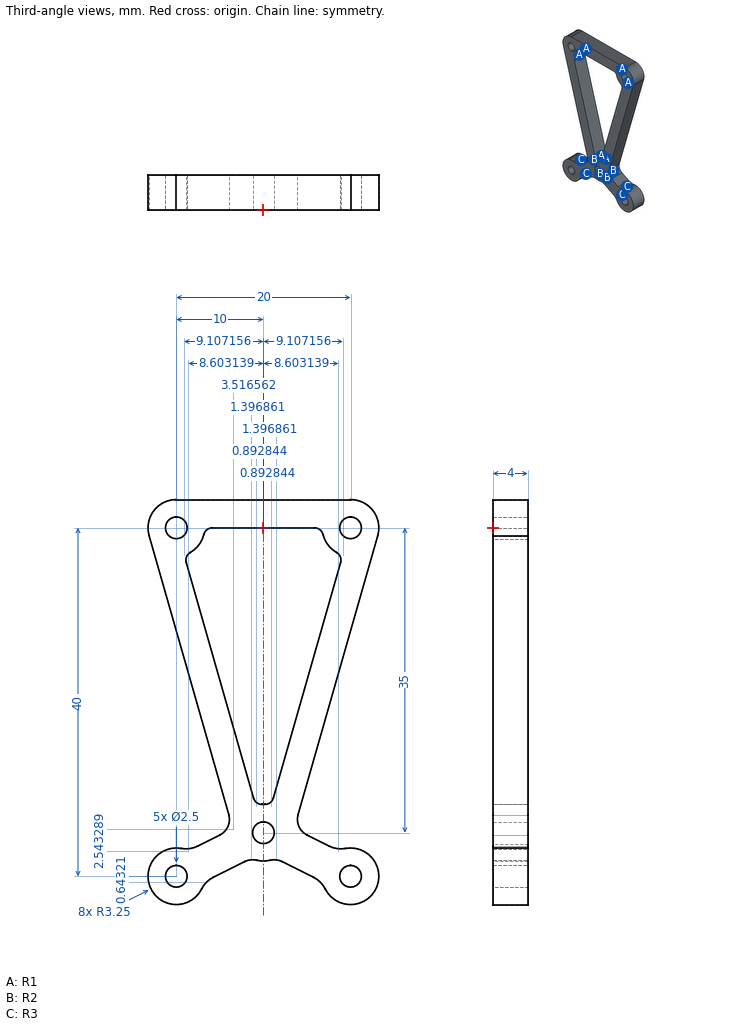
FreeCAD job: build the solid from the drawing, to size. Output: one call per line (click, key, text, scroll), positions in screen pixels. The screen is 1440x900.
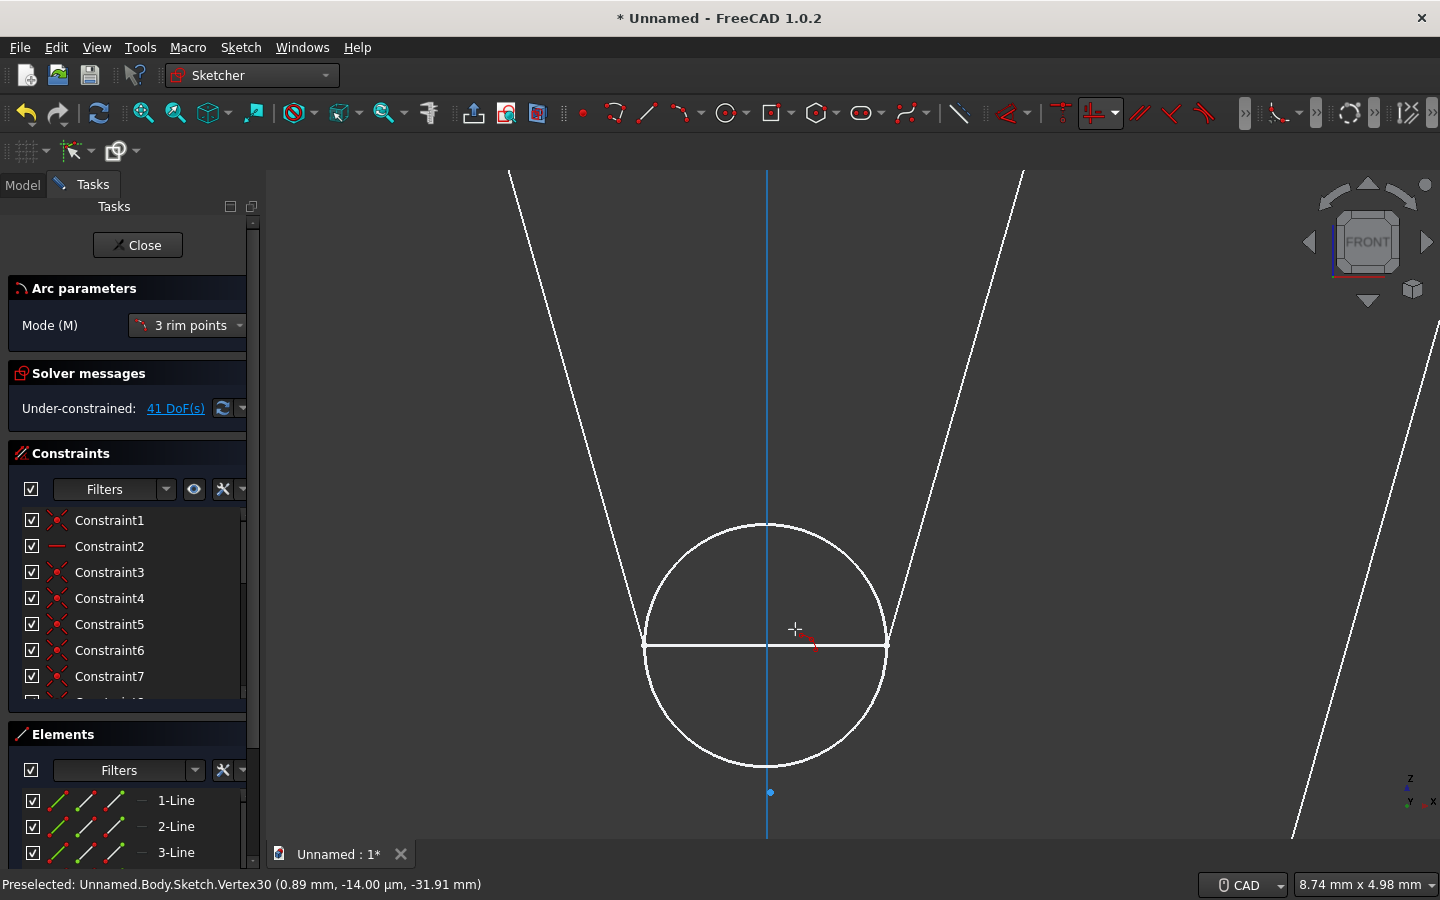
click(792, 624)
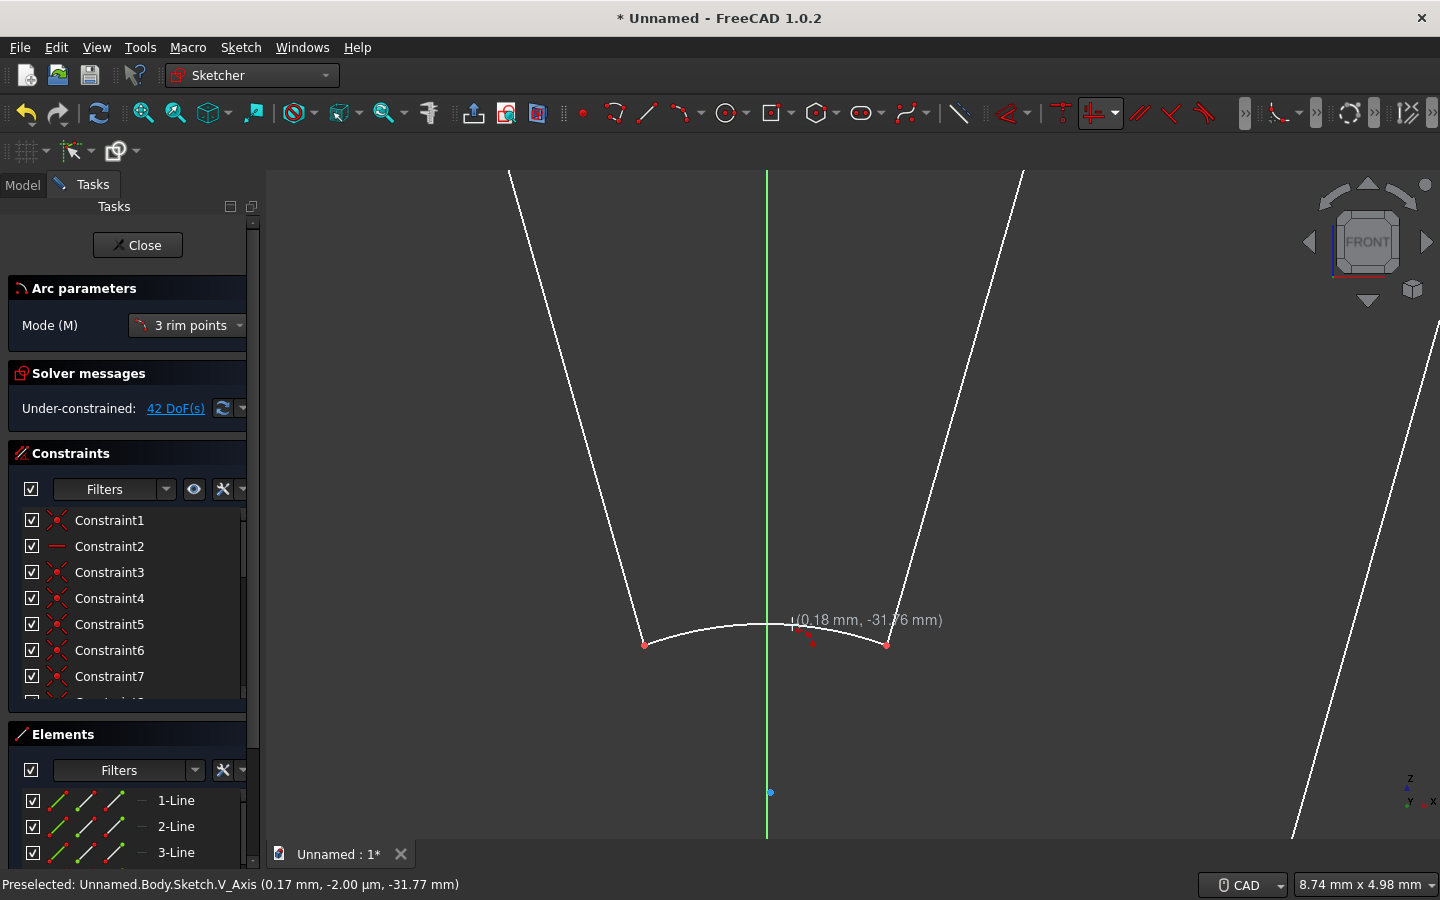
key(g)
key(c)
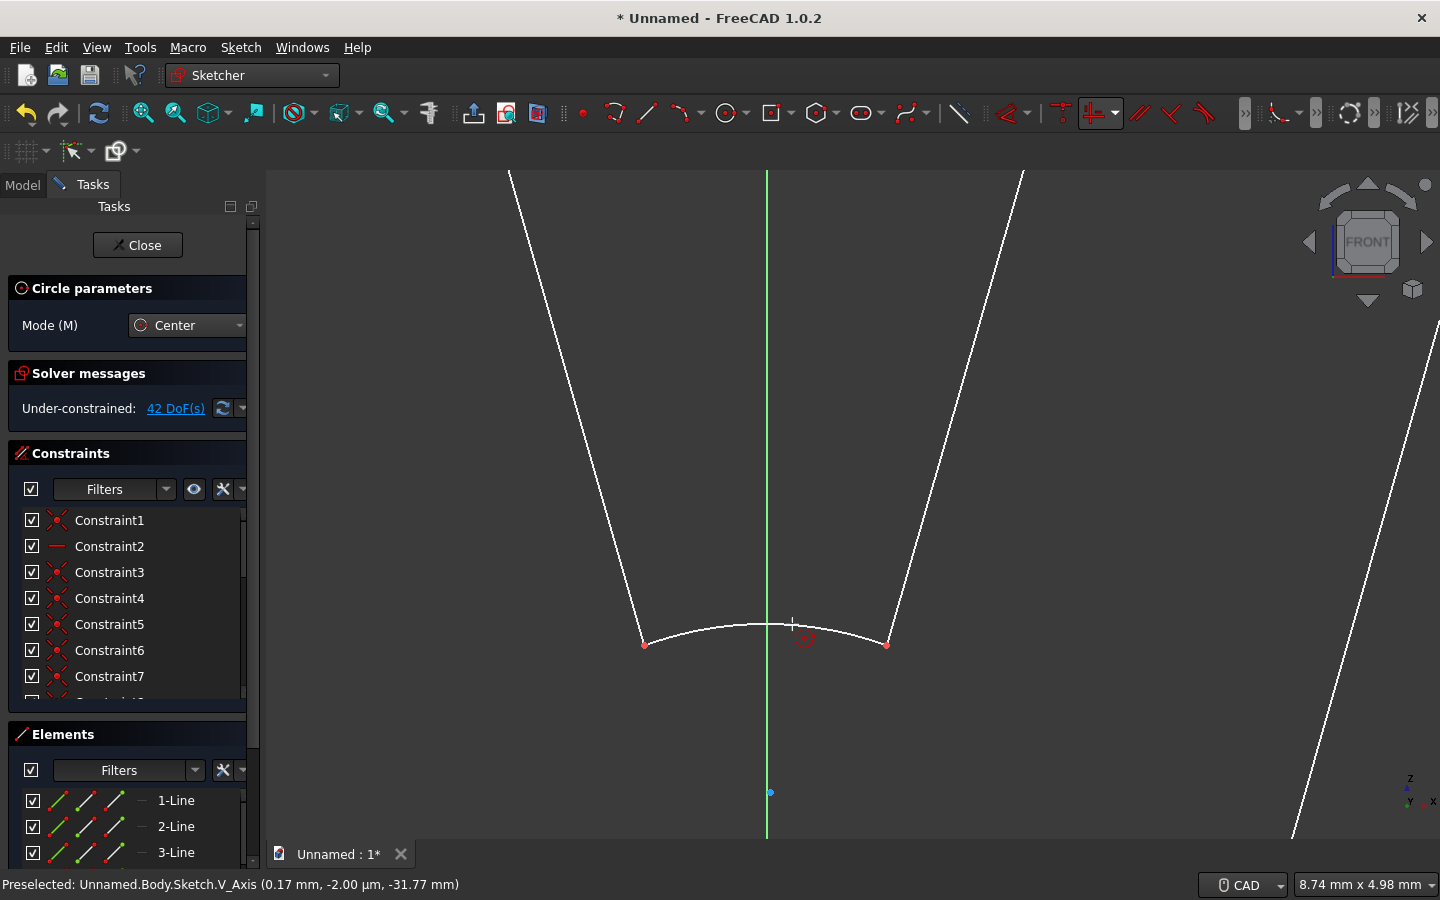
scroll(786, 631, down, 13)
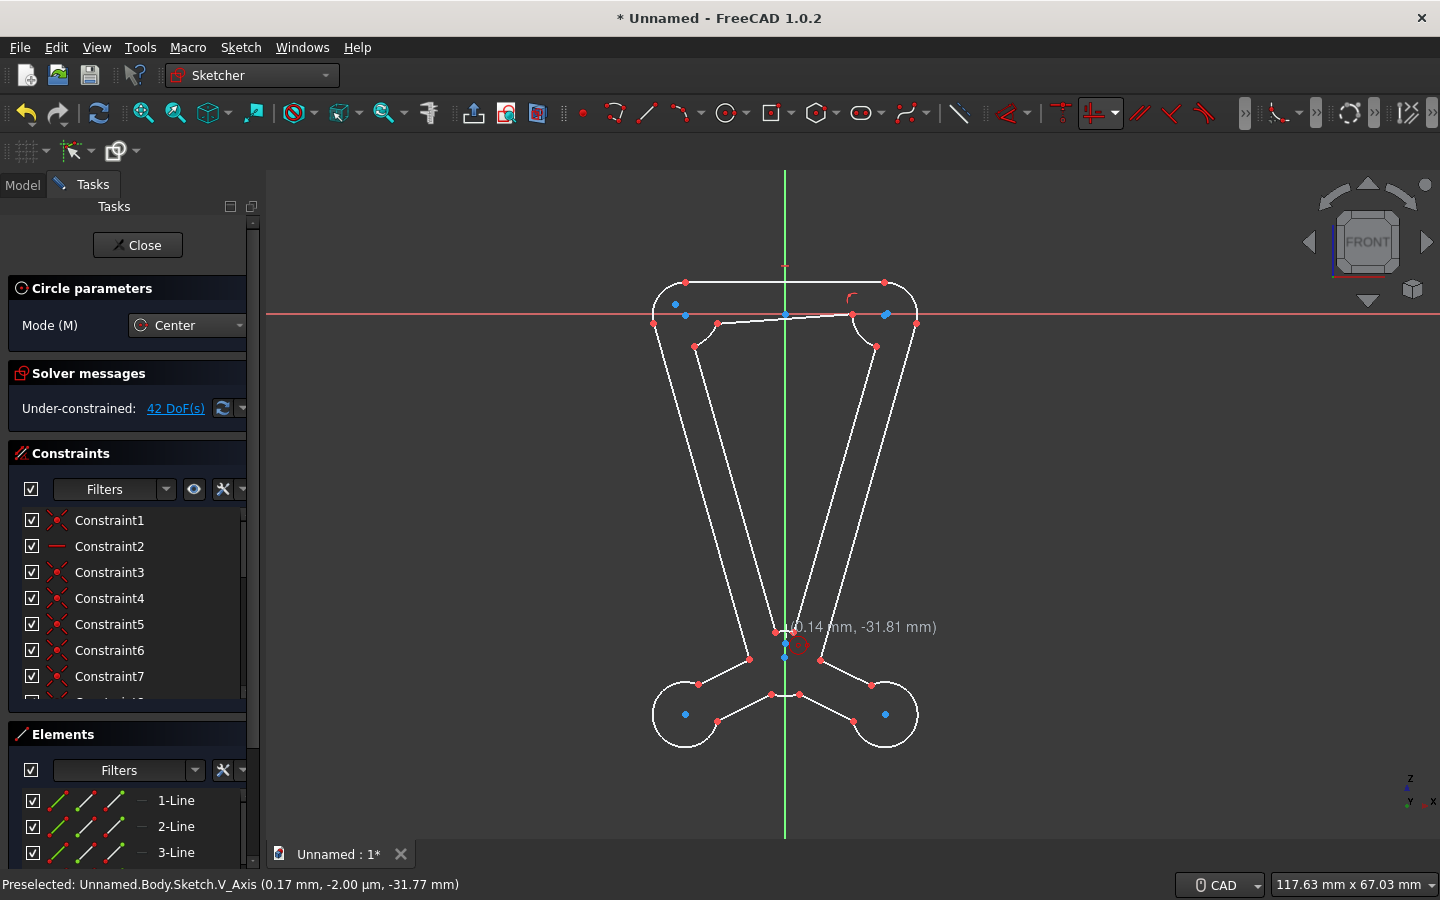
scroll(685, 713, up, 3)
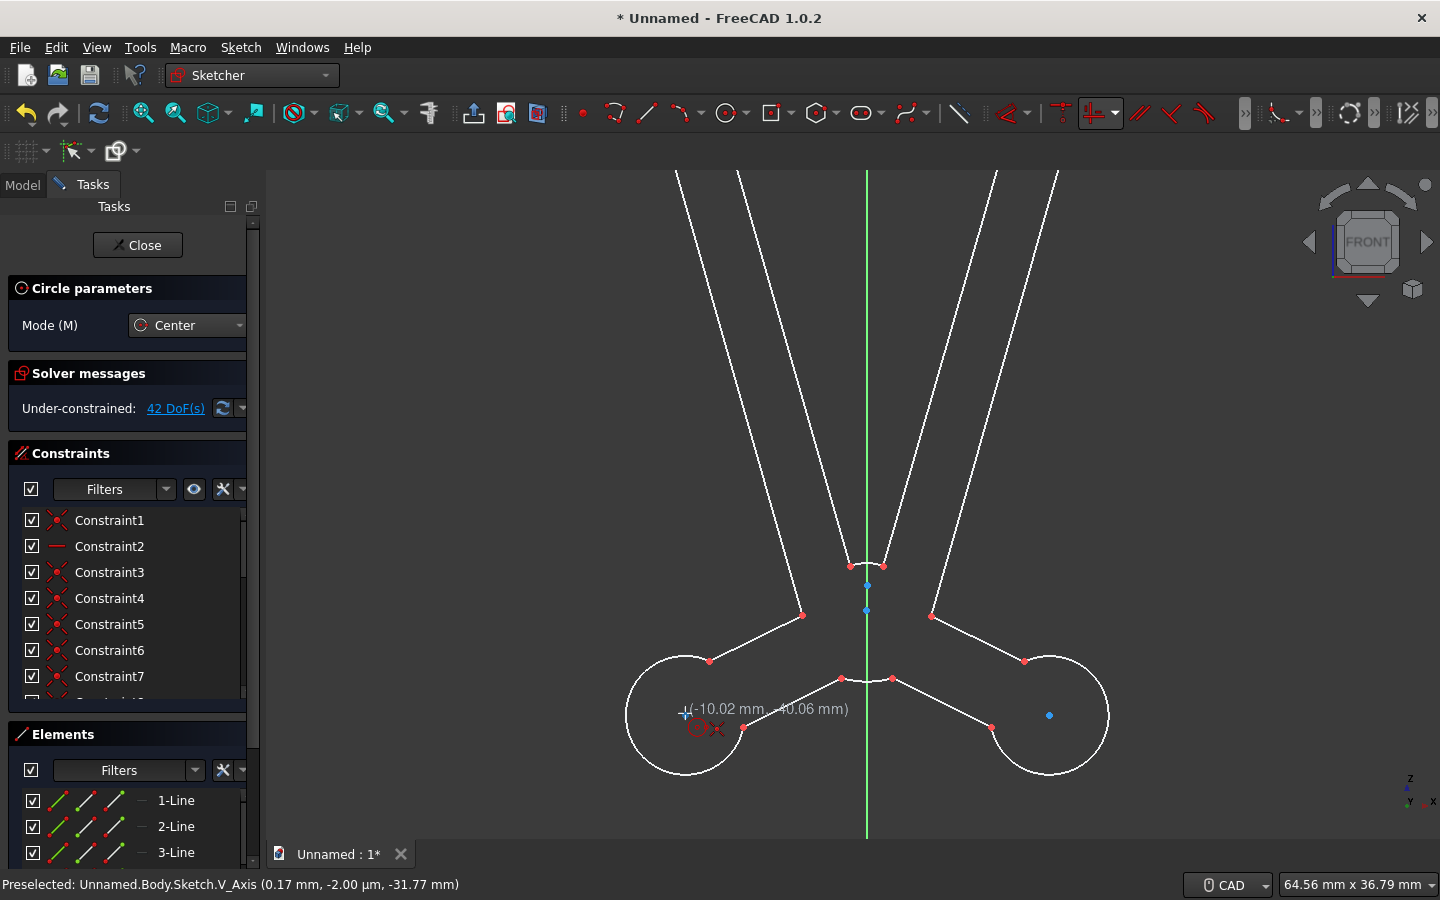
click(685, 713)
move(701, 697)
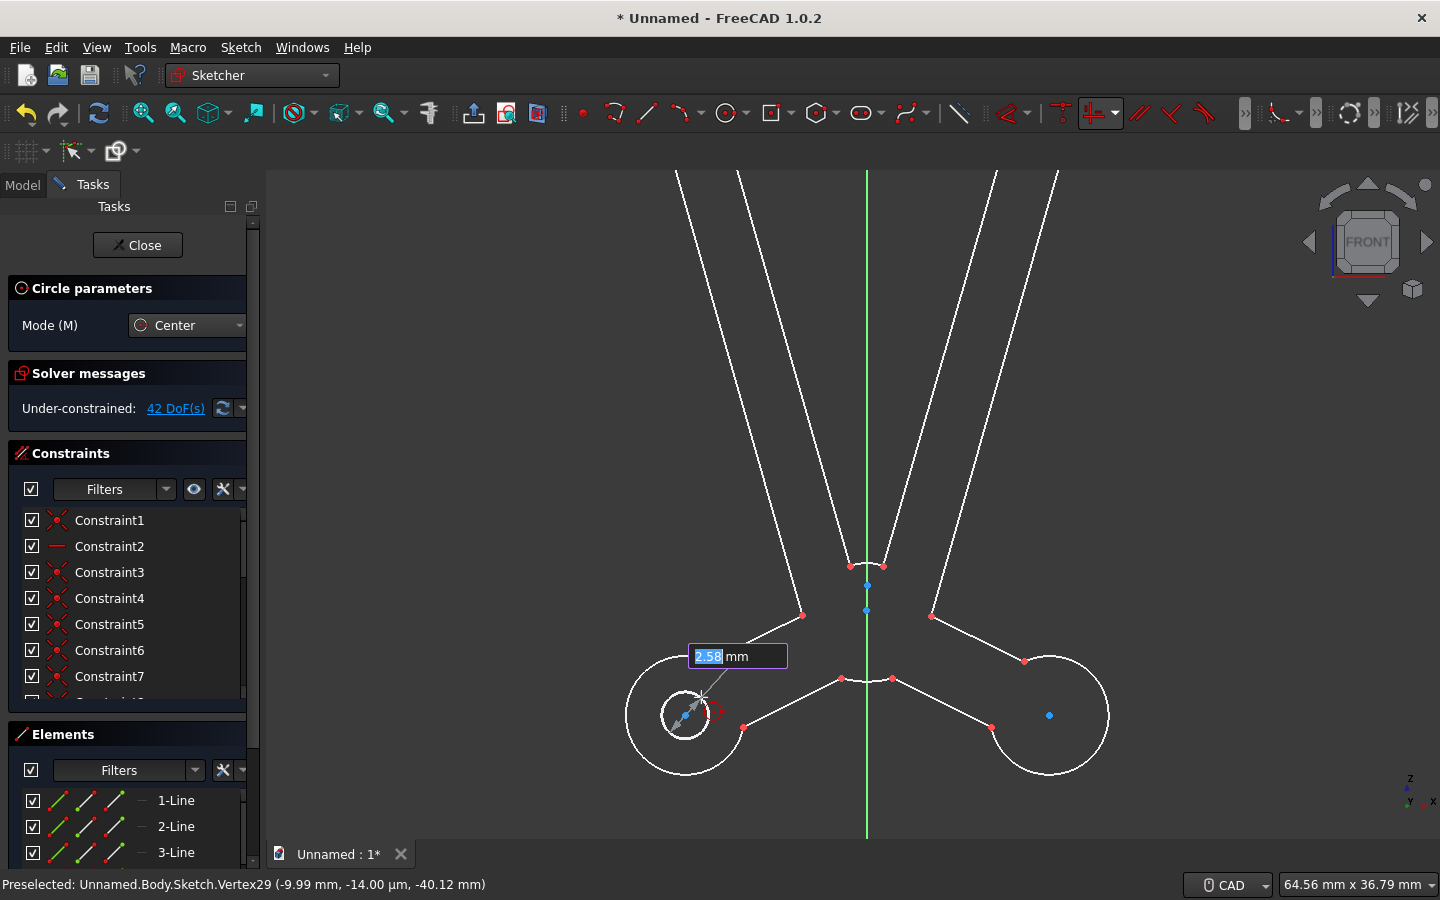
text(2.5)
key(Return)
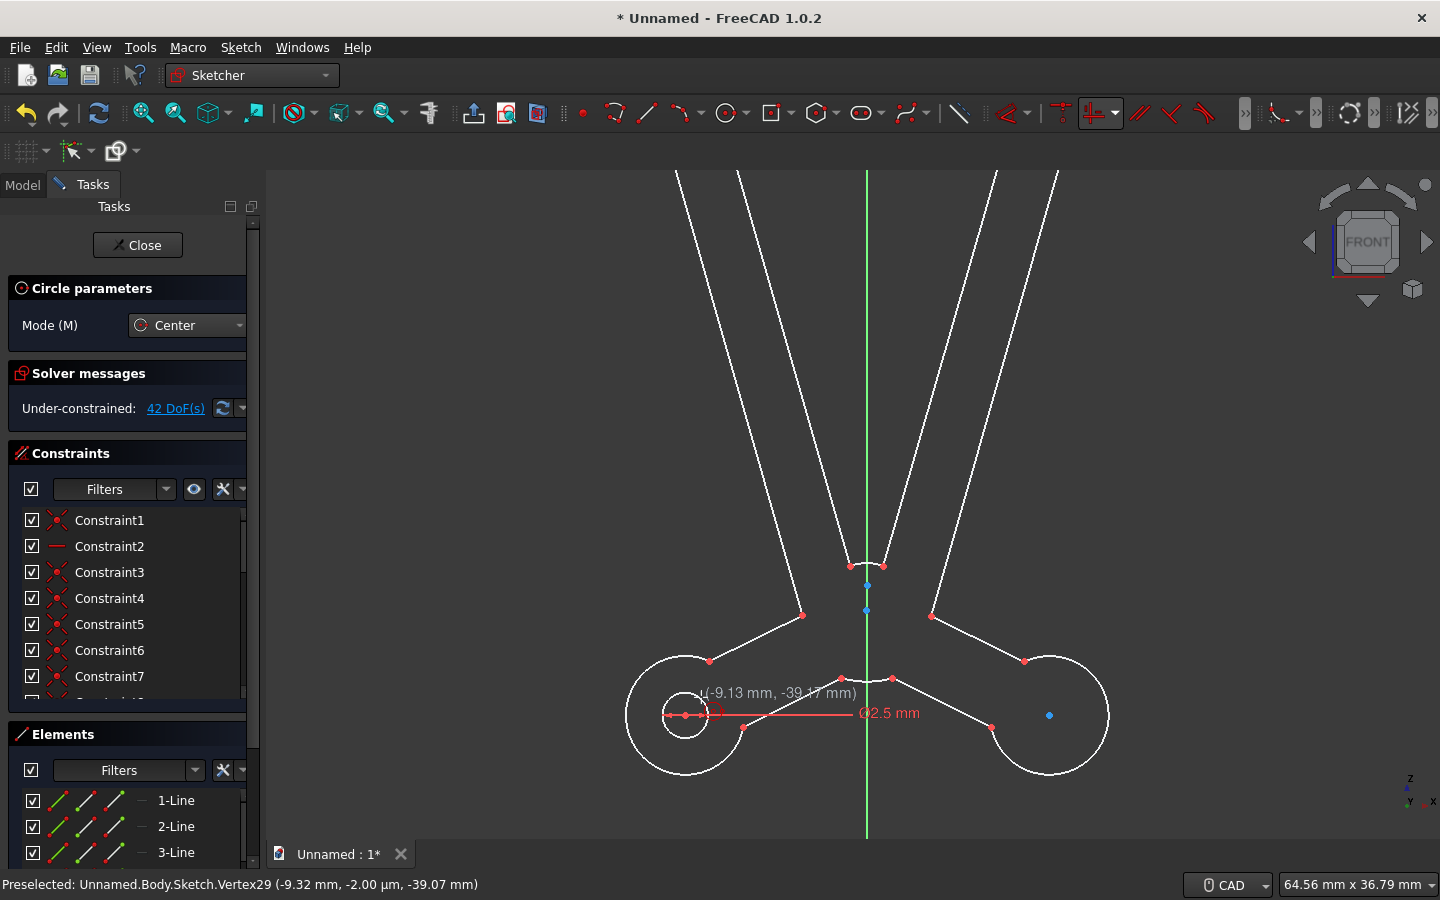
click(867, 622)
move(883, 606)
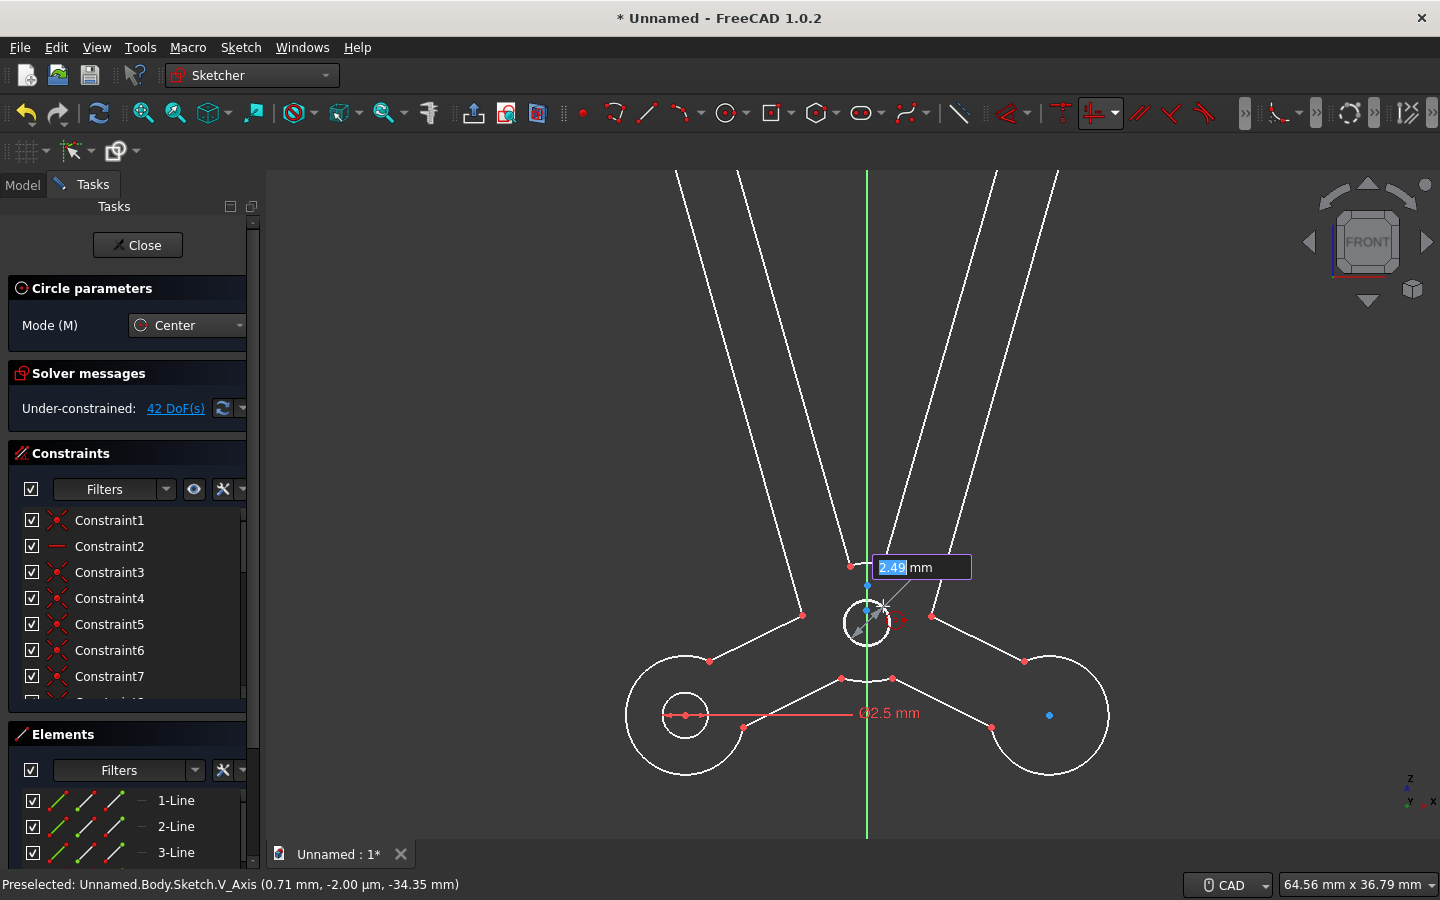
text(2.5)
key(Return)